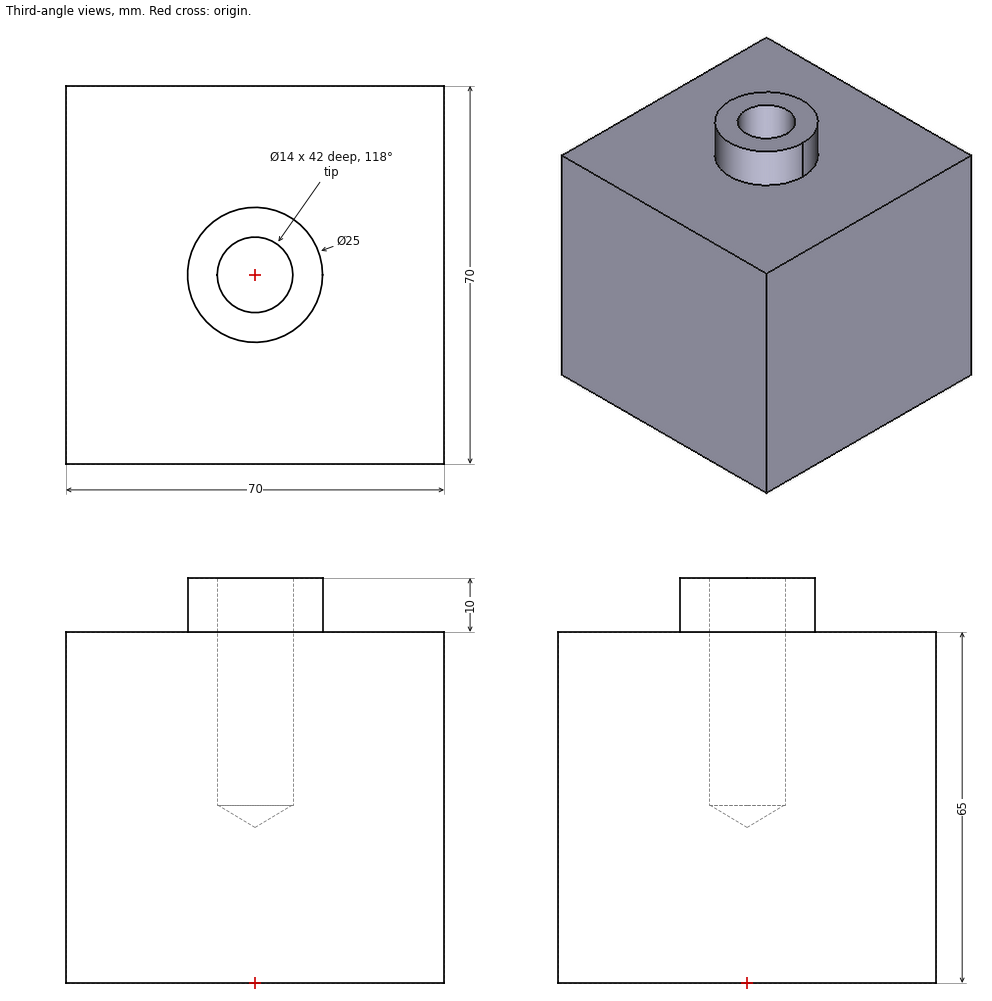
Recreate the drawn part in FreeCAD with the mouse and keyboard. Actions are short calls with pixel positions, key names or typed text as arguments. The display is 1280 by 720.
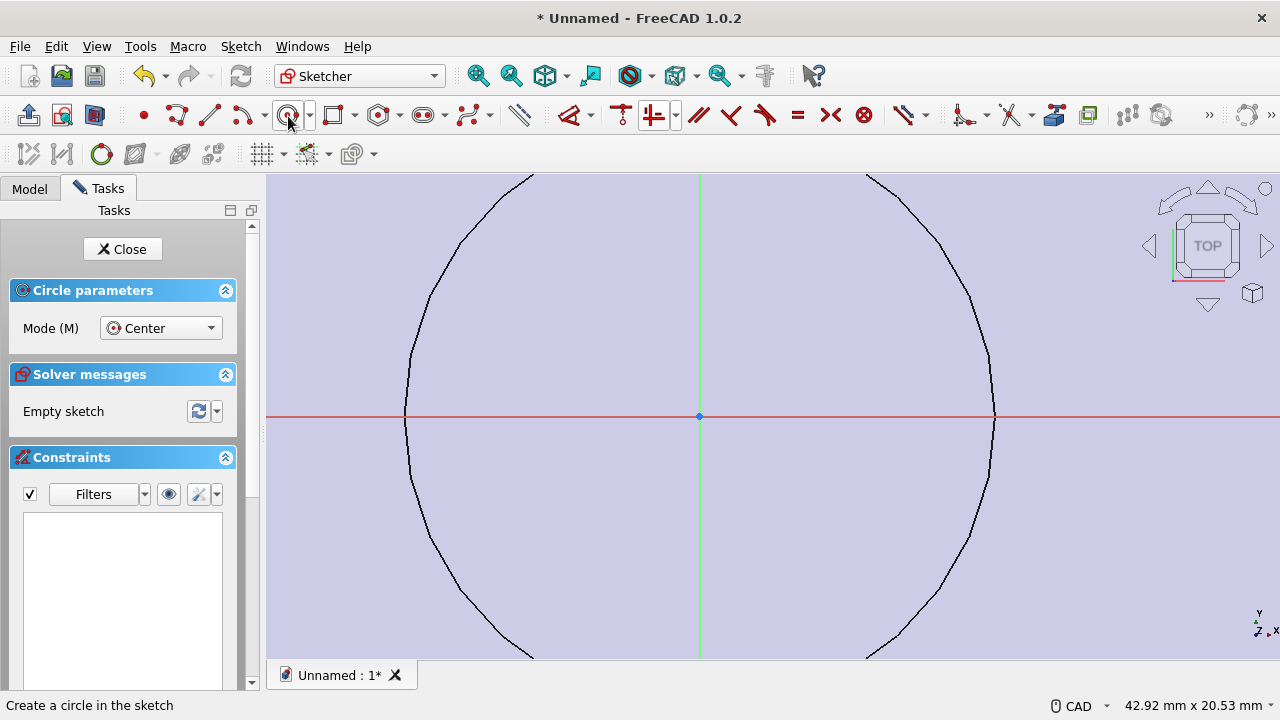
click(700, 416)
click(817, 300)
key(Escape)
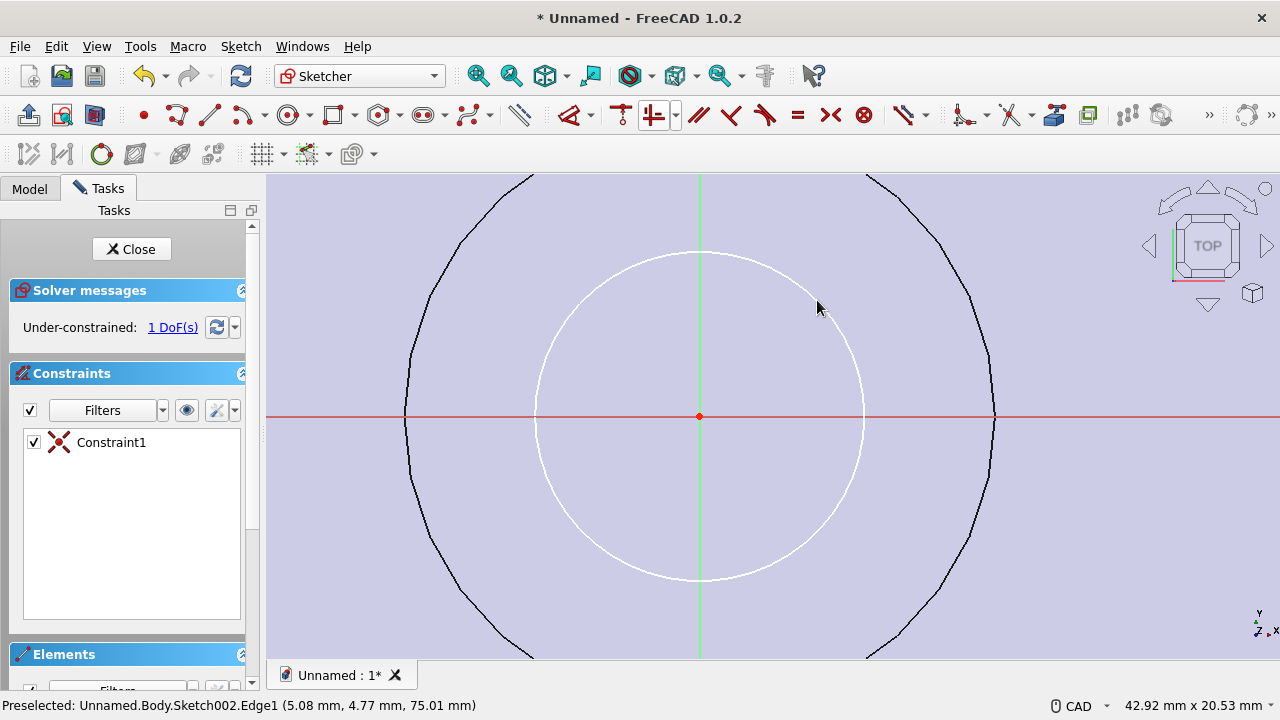
click(568, 116)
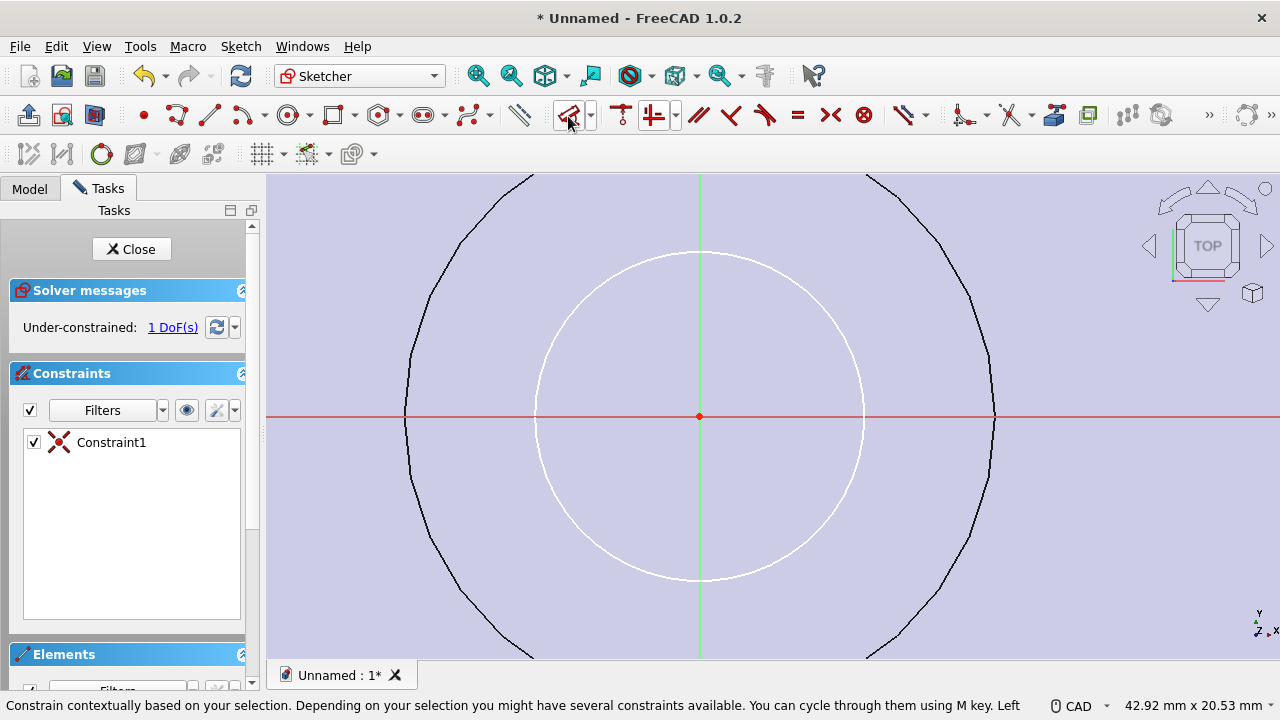
click(816, 300)
click(839, 277)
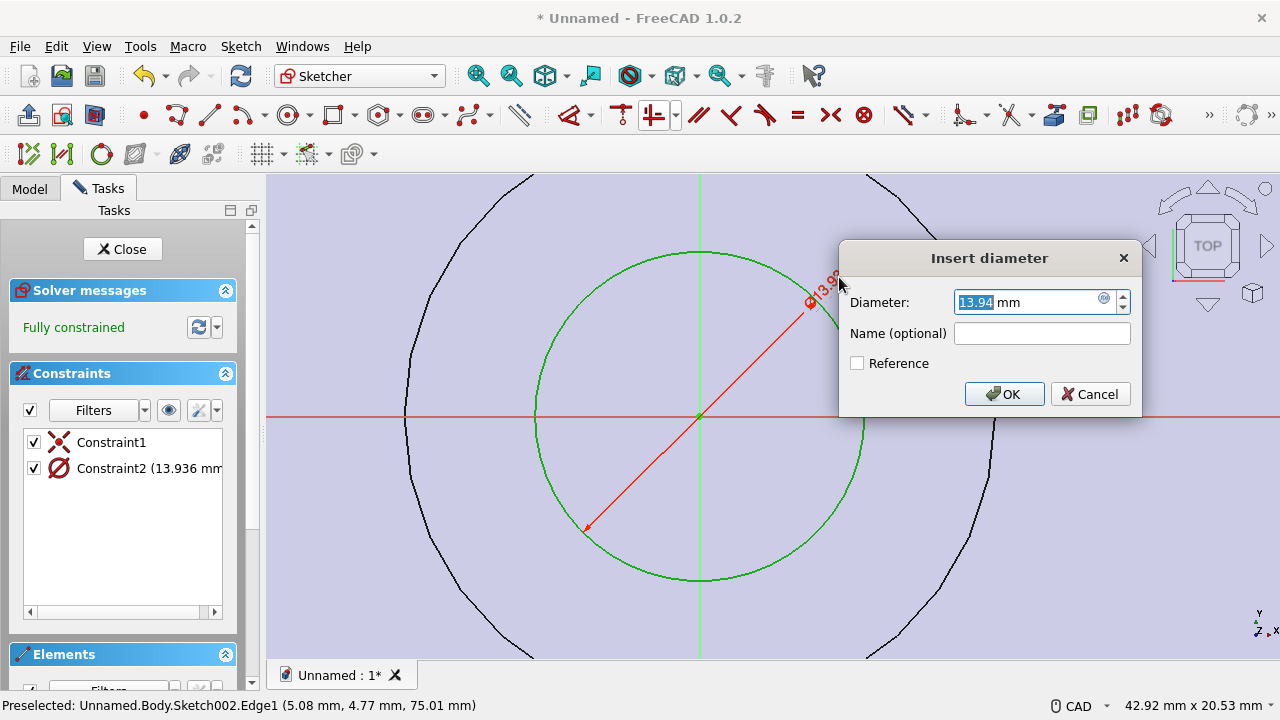
text(14)
key(Return)
key(Escape)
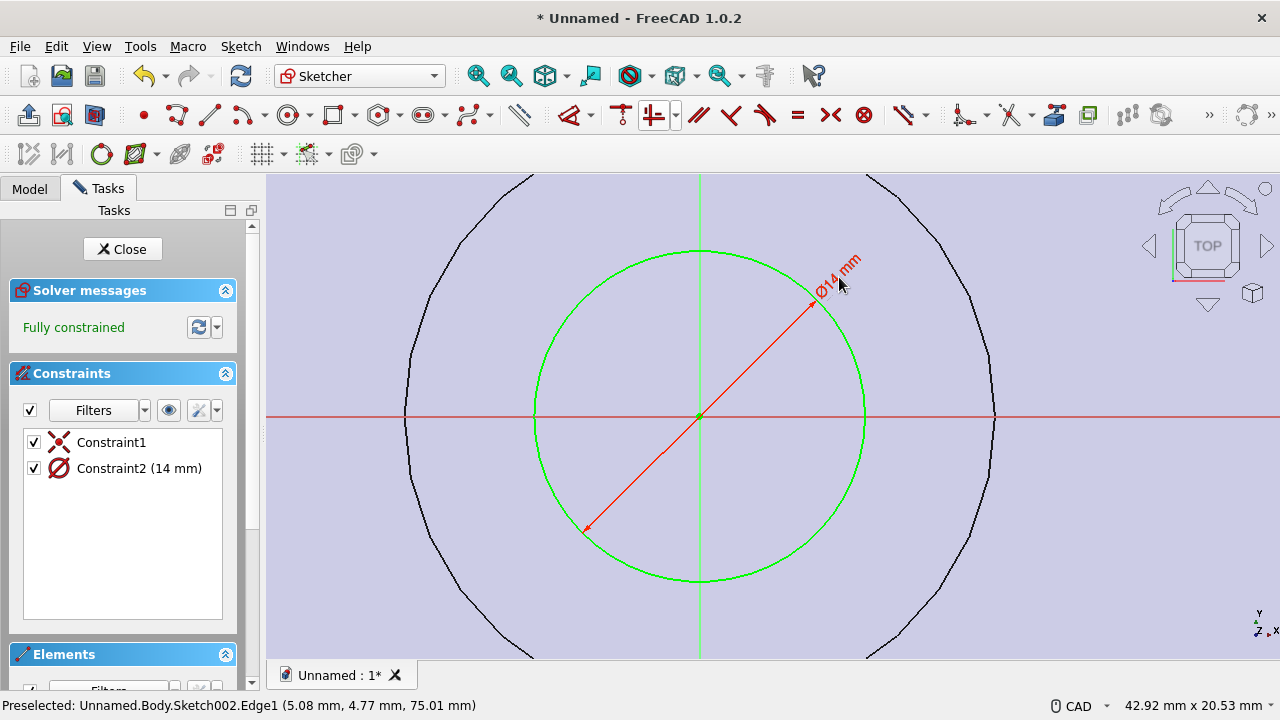
click(123, 249)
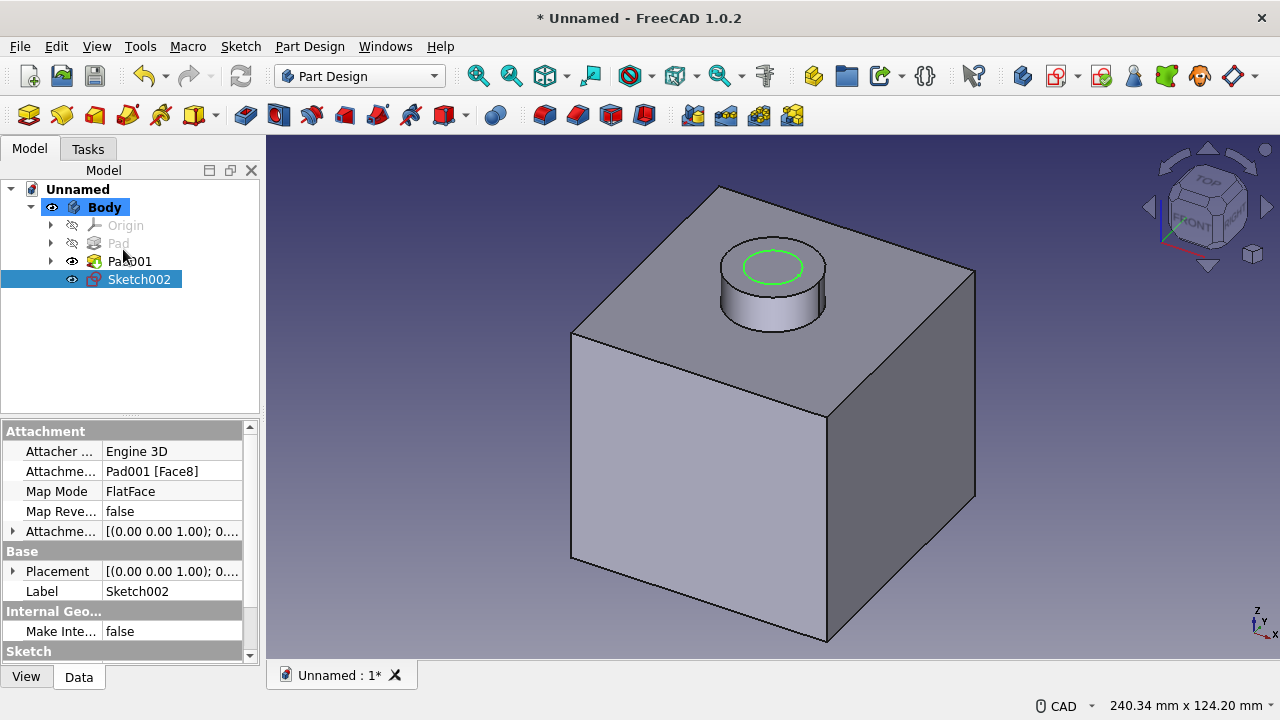
click(279, 116)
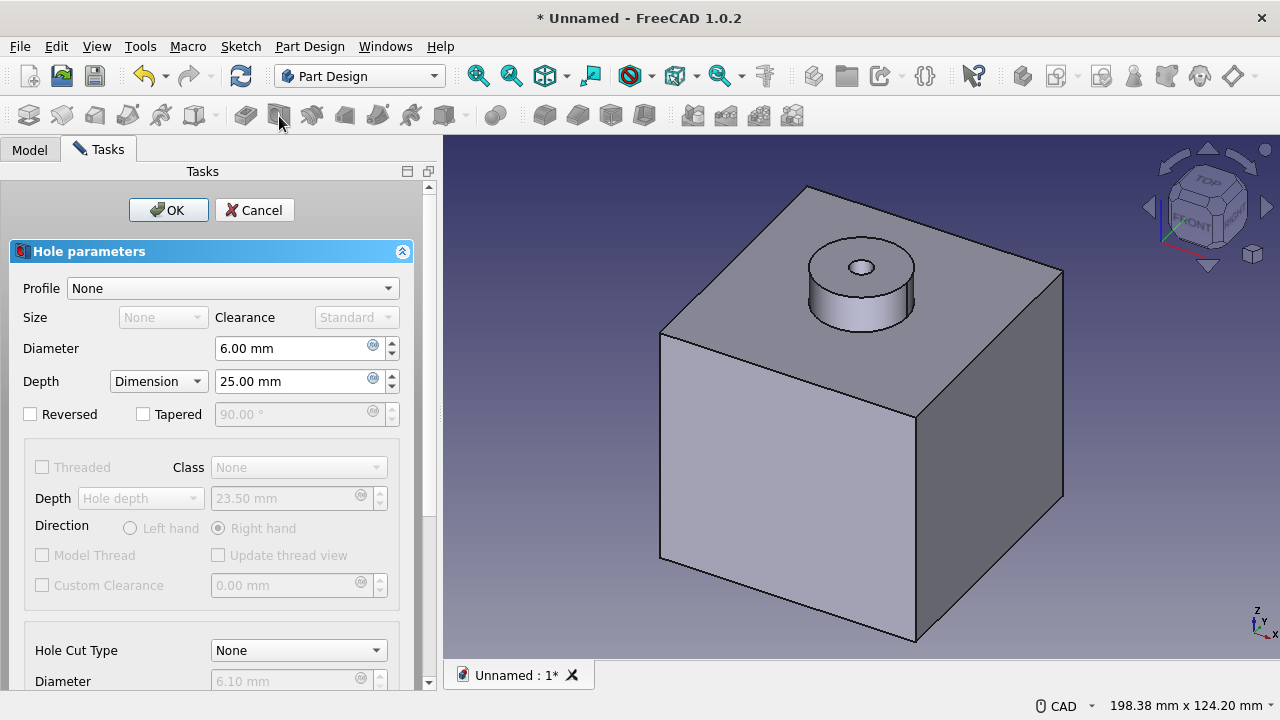
triple_click(300, 348)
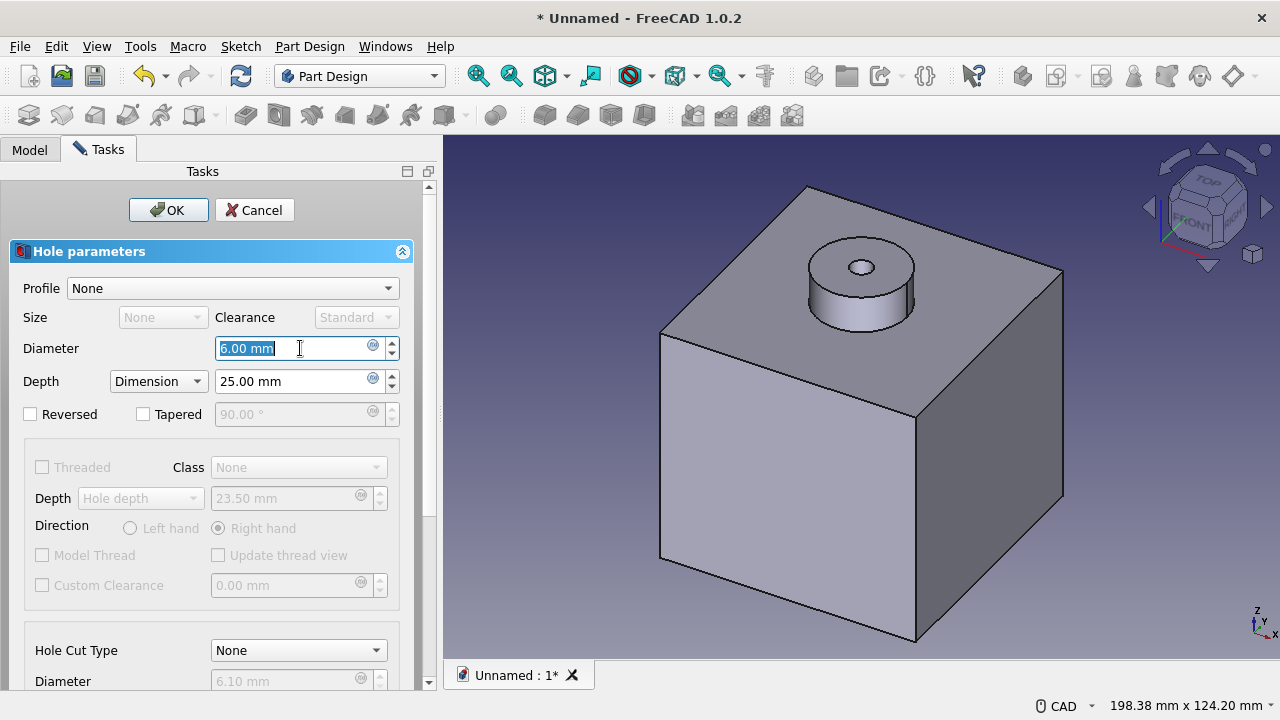
text(14)
key(Tab)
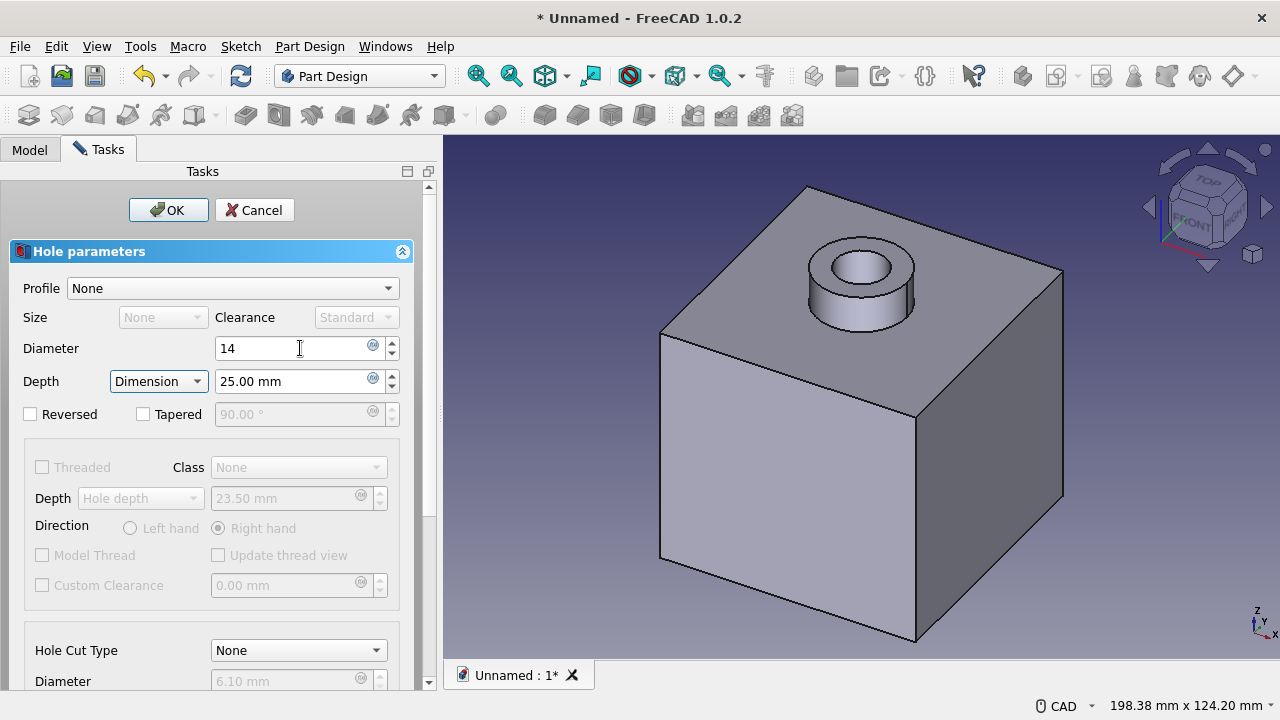
triple_click(300, 382)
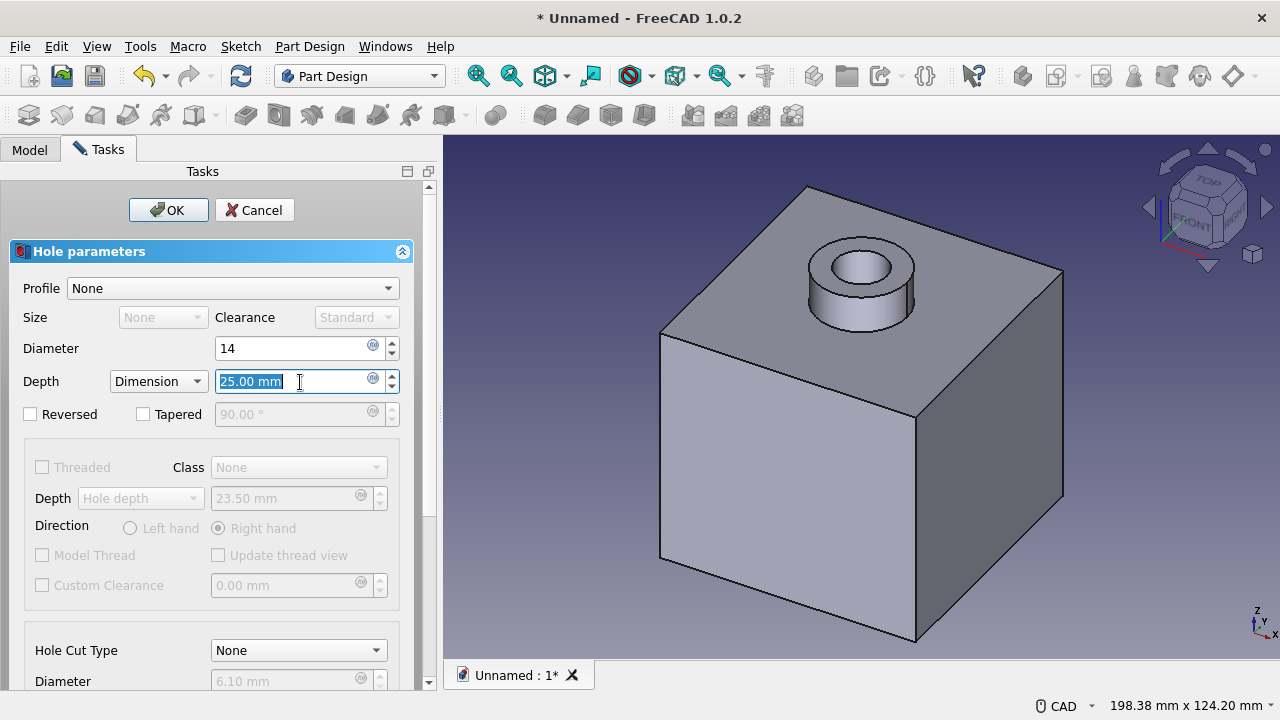
text(42)
key(Tab)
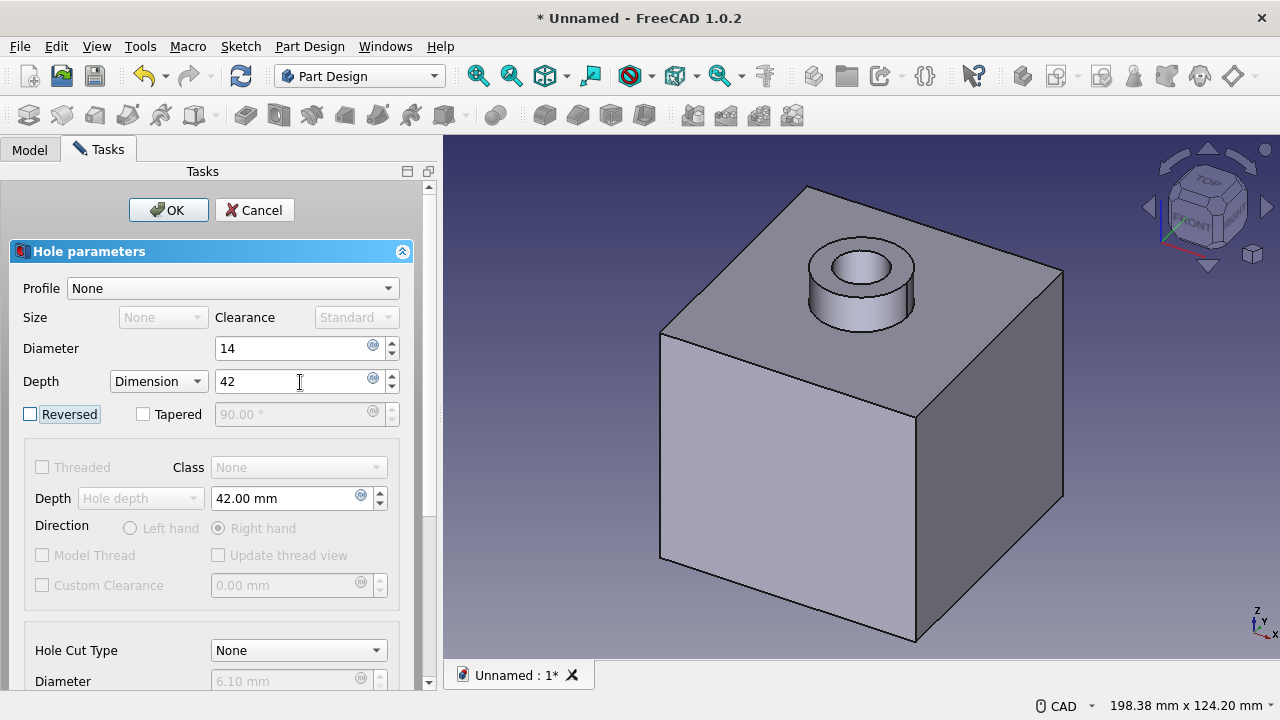
click(169, 210)